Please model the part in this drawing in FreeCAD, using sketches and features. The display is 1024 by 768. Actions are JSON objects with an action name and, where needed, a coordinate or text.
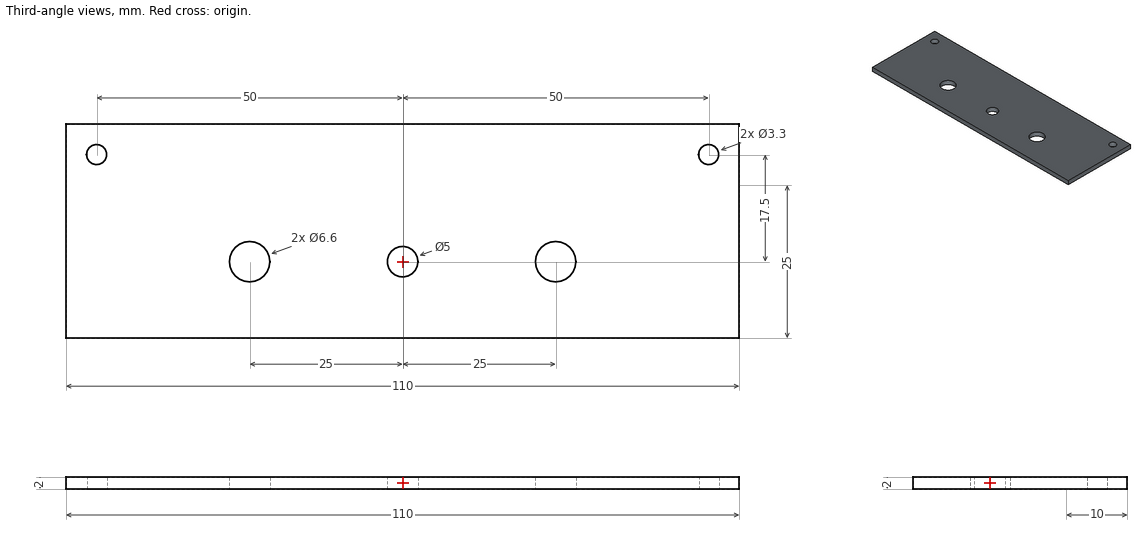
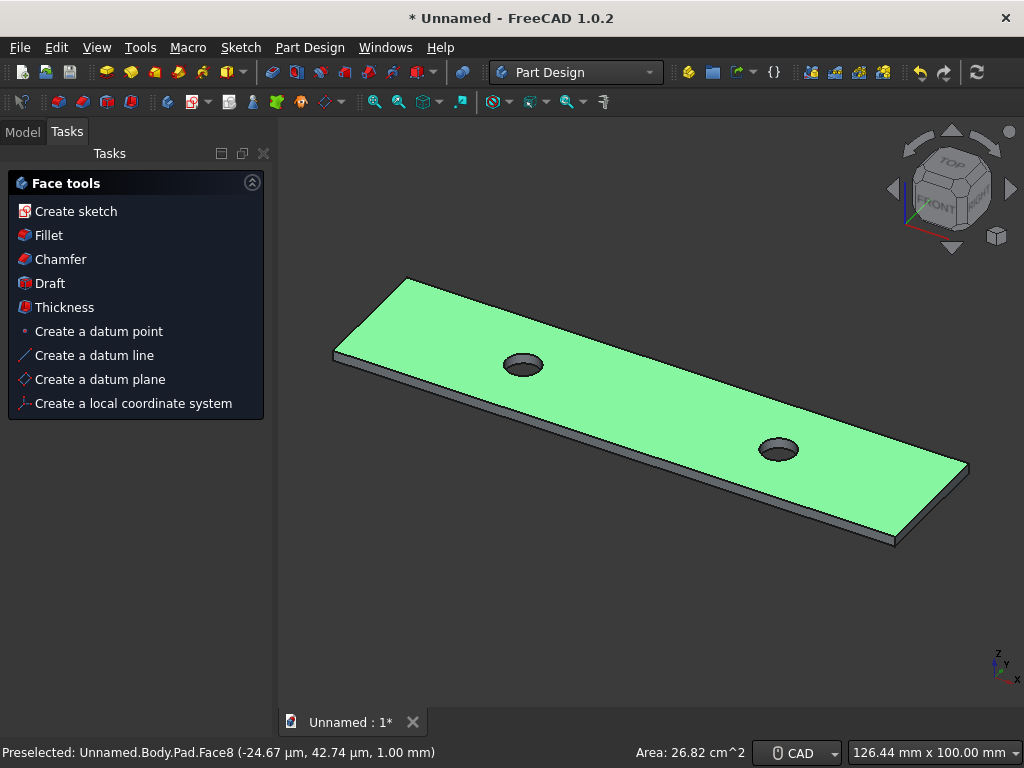
{"action": "left_click", "coordinate": [192, 102]}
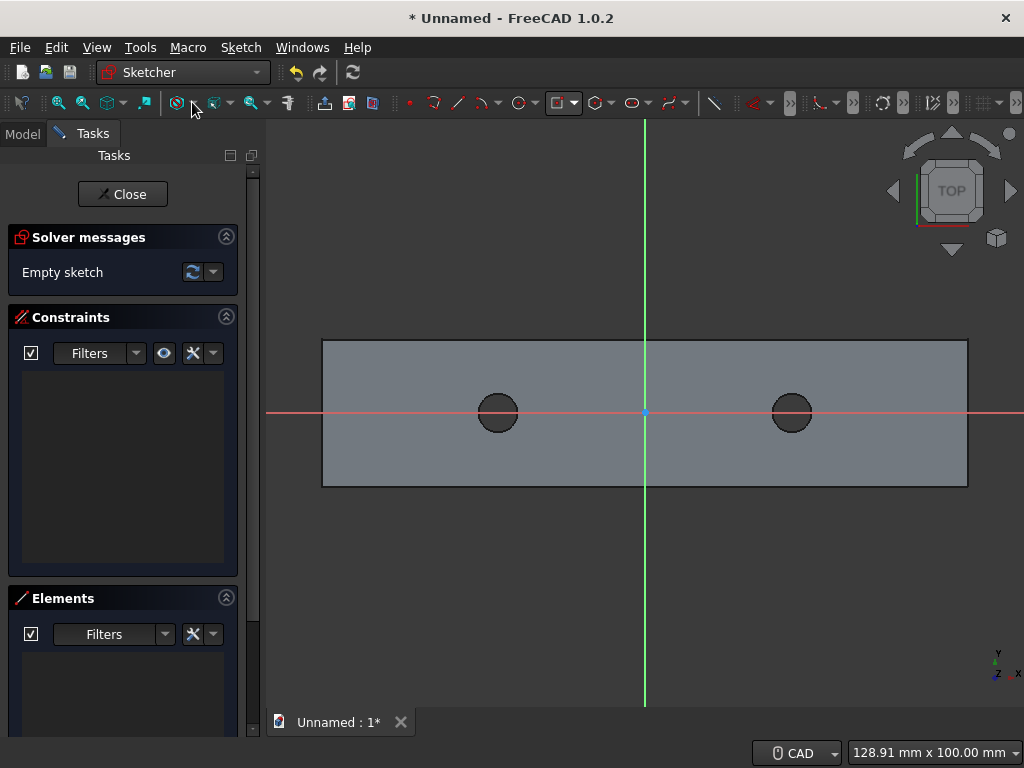
{"action": "scroll", "coordinate": [650, 413], "scroll_direction": "up", "scroll_amount": 13}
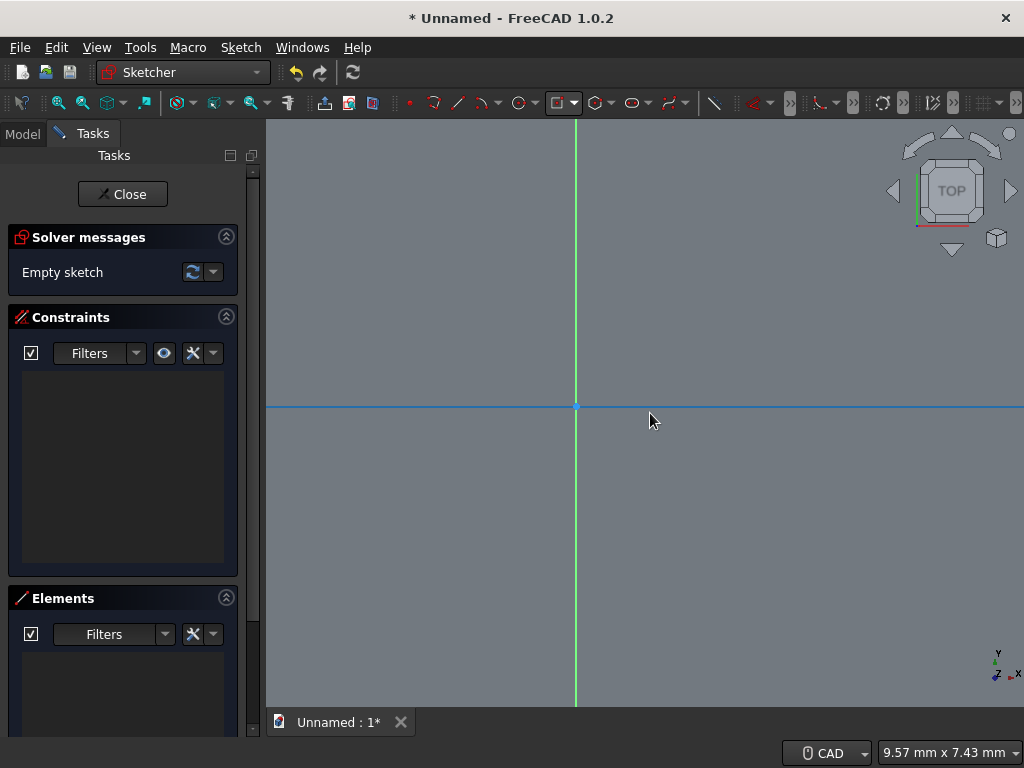
{"action": "key", "text": "g c"}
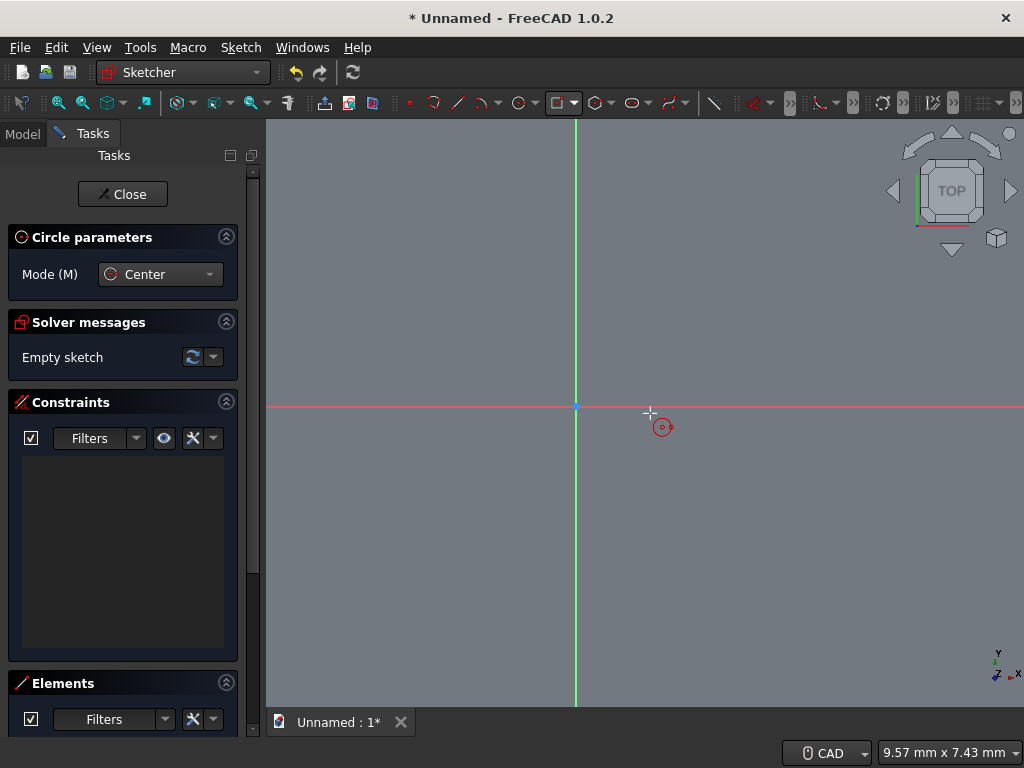
{"action": "left_click", "coordinate": [576, 407]}
{"action": "mouse_move", "coordinate": [716, 267]}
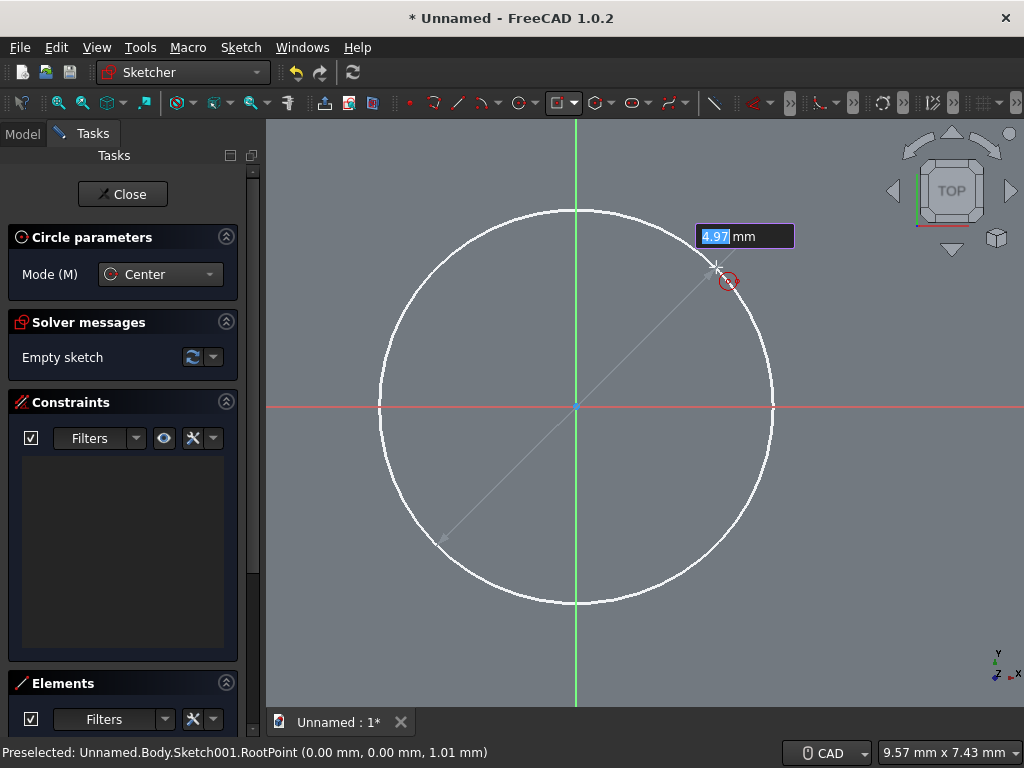
{"action": "type", "text": "5"}
{"action": "key", "text": "Return"}
{"action": "key", "text": "Escape"}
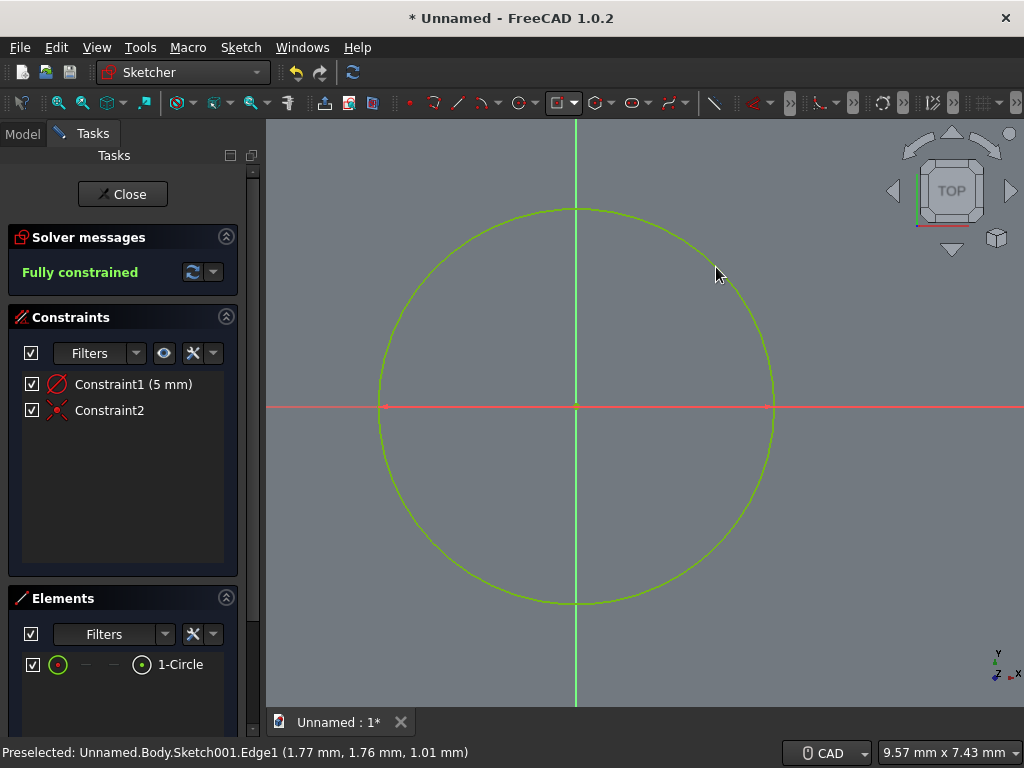
{"action": "left_click", "coordinate": [123, 194]}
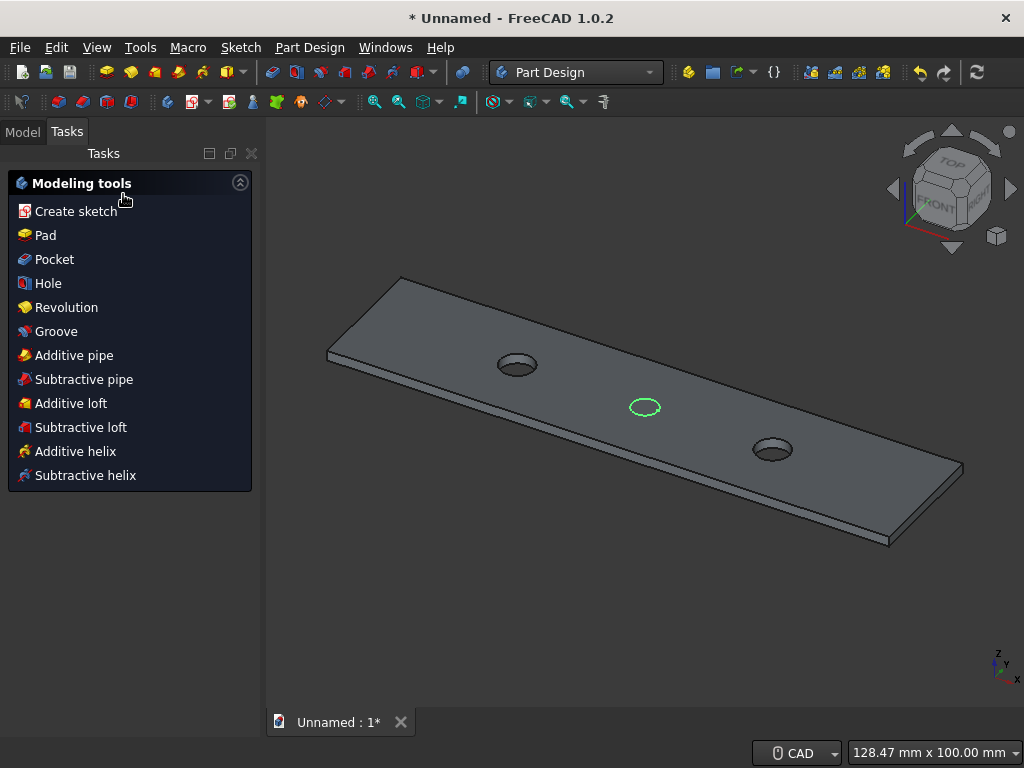
{"action": "left_click", "coordinate": [274, 72]}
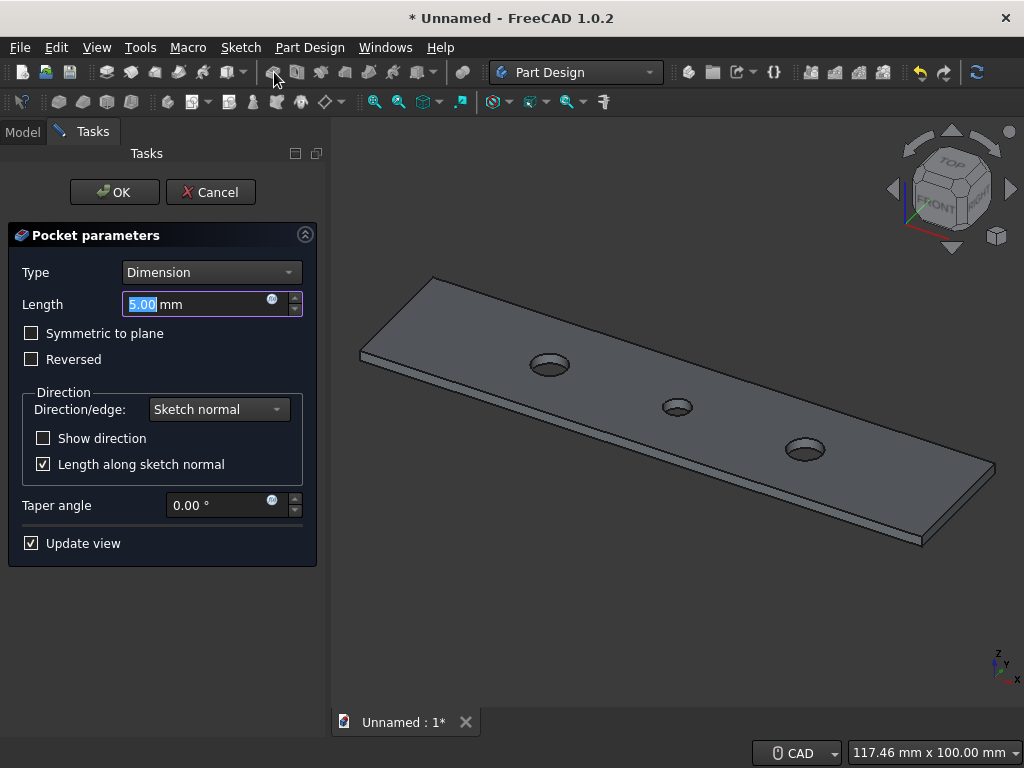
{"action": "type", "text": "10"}
{"action": "key", "text": "Tab"}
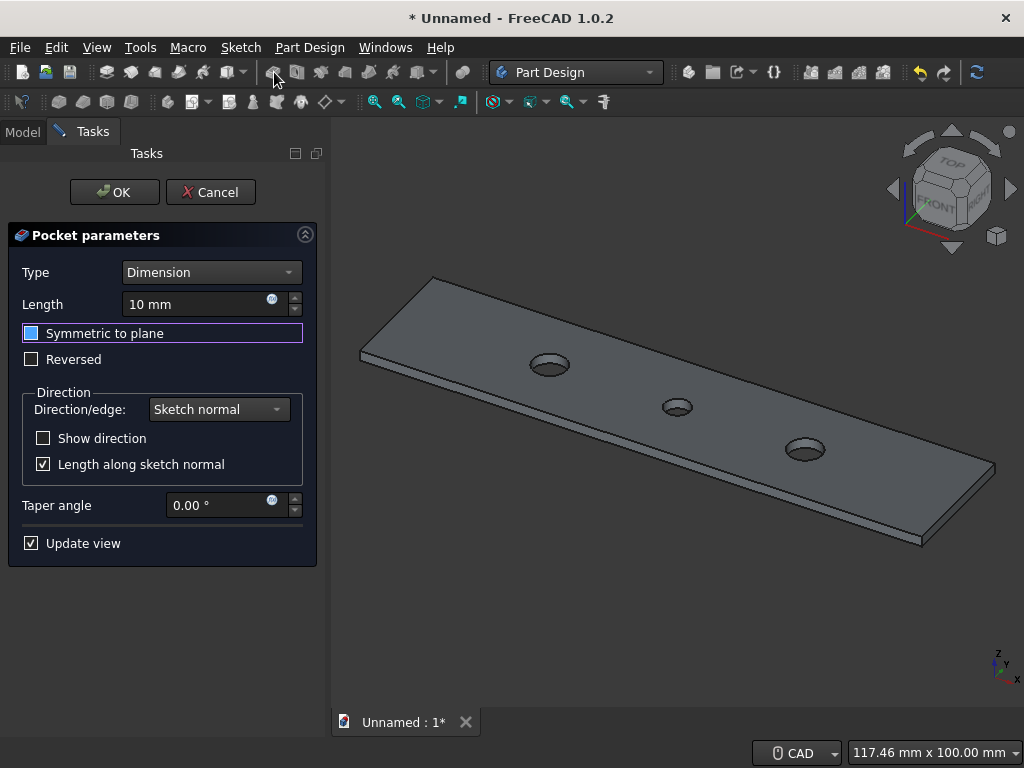
{"action": "left_click", "coordinate": [115, 192]}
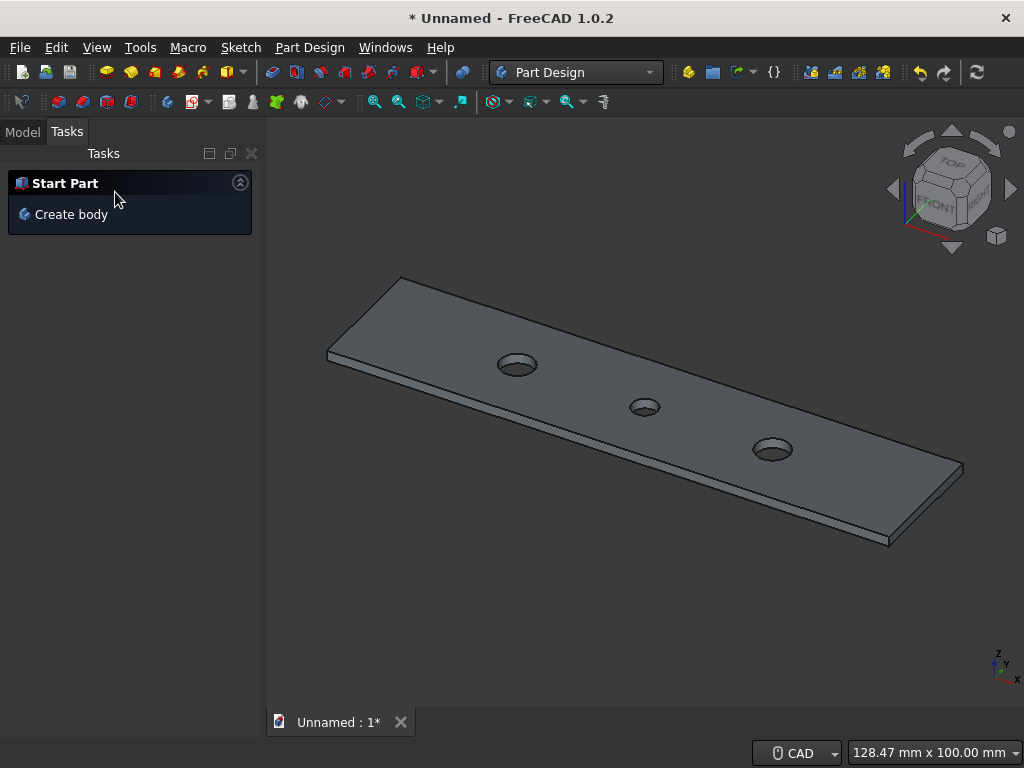
{"action": "key", "text": "4"}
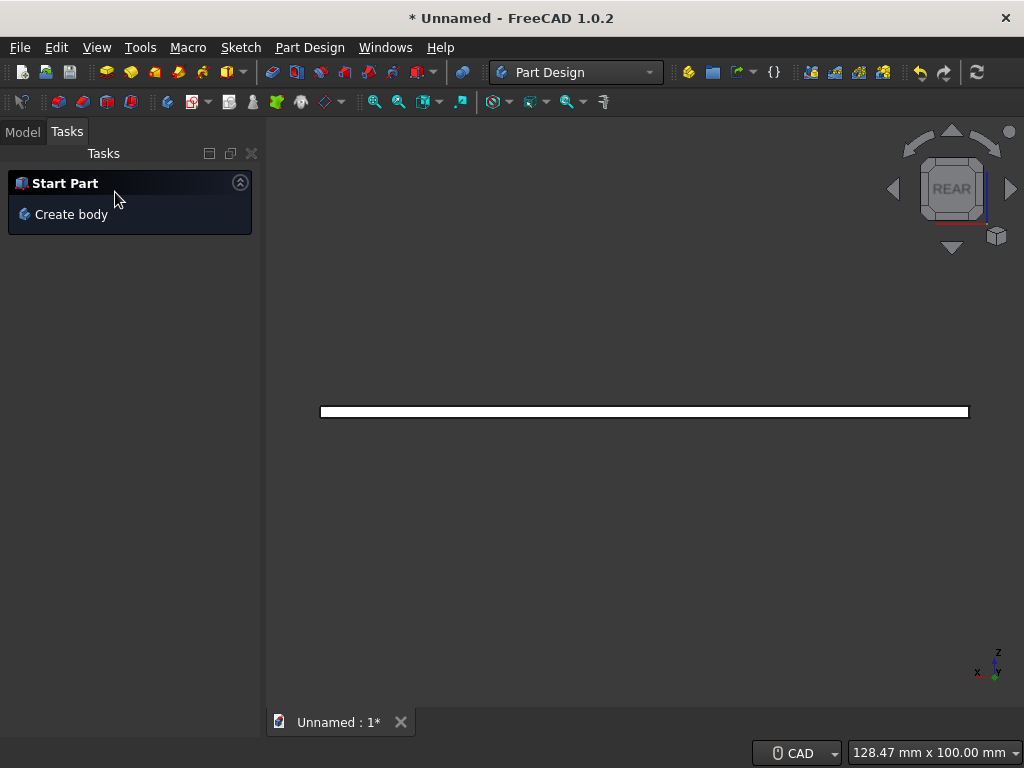
{"action": "scroll", "coordinate": [367, 411], "scroll_direction": "up", "scroll_amount": 4}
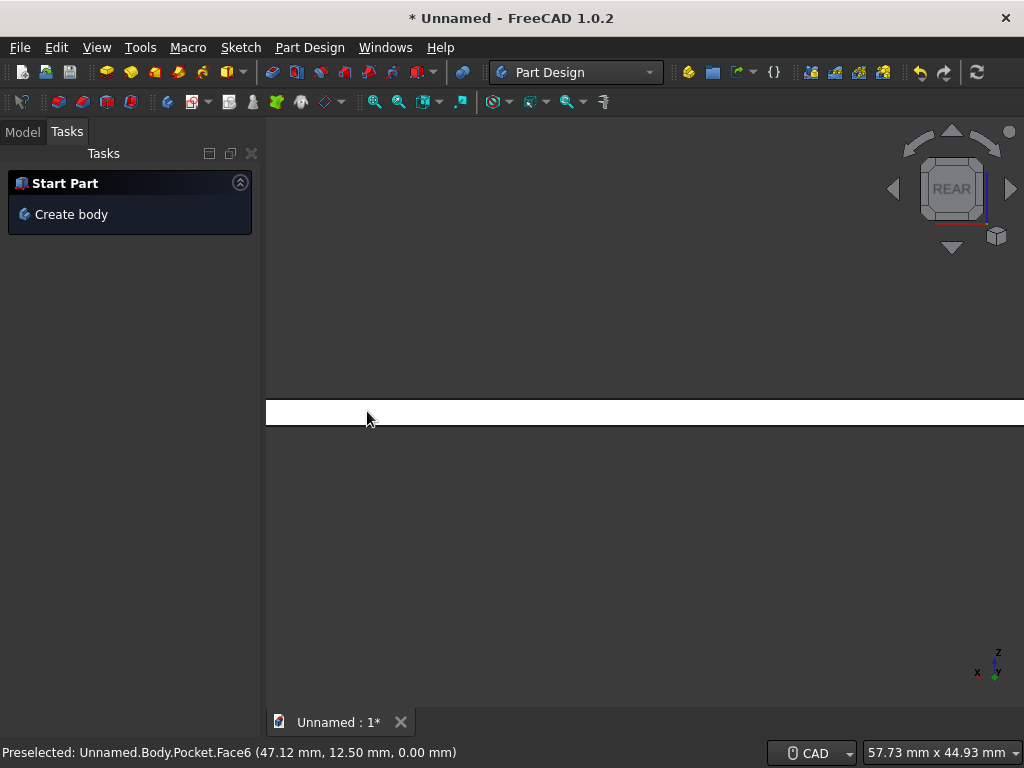
{"action": "left_click", "coordinate": [367, 412]}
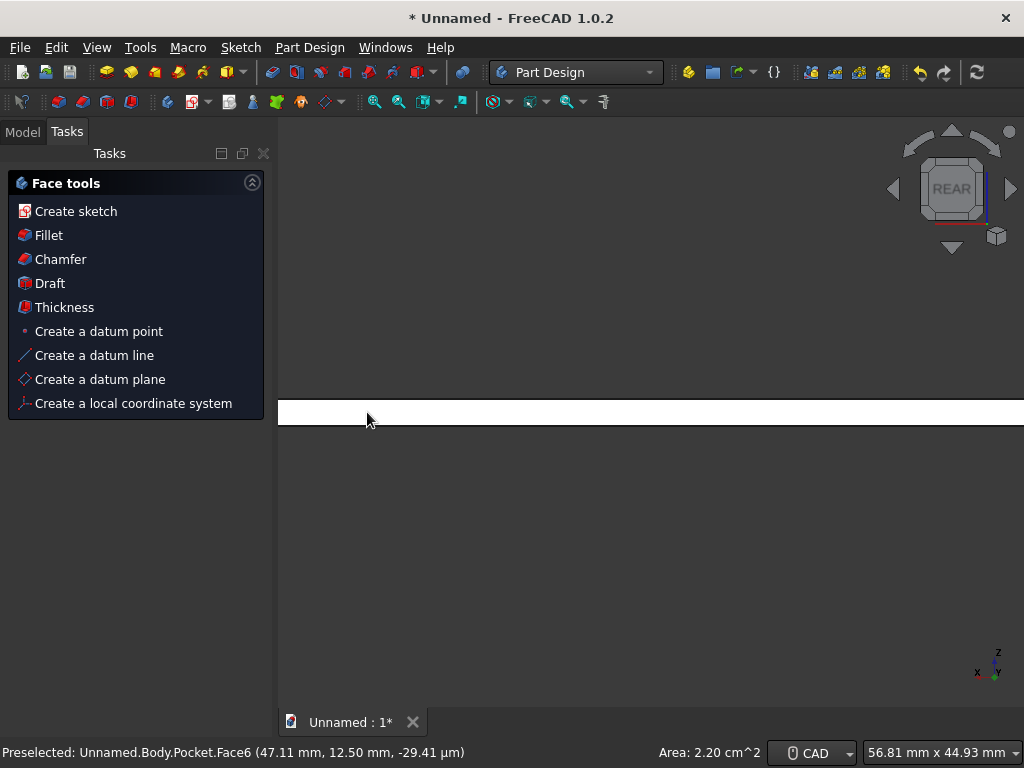
{"action": "left_click", "coordinate": [192, 102]}